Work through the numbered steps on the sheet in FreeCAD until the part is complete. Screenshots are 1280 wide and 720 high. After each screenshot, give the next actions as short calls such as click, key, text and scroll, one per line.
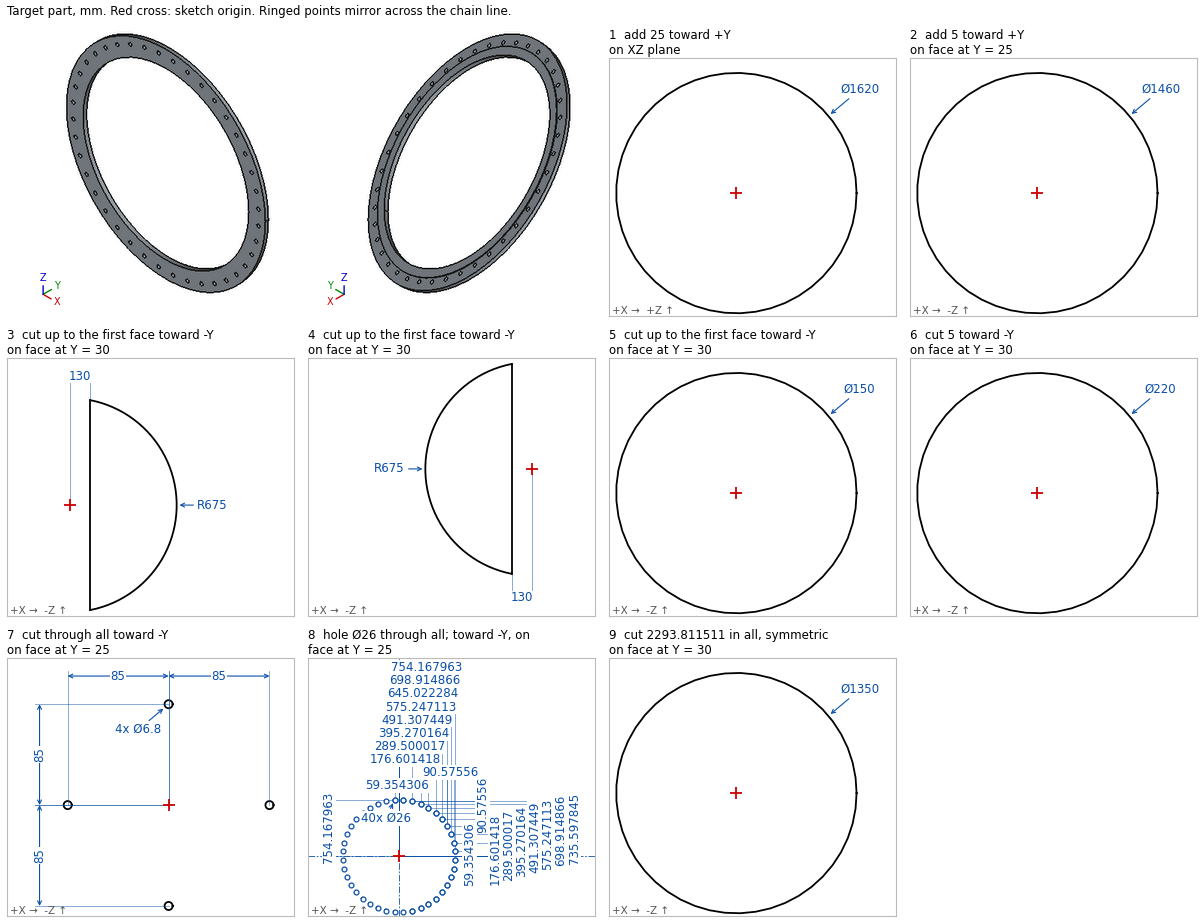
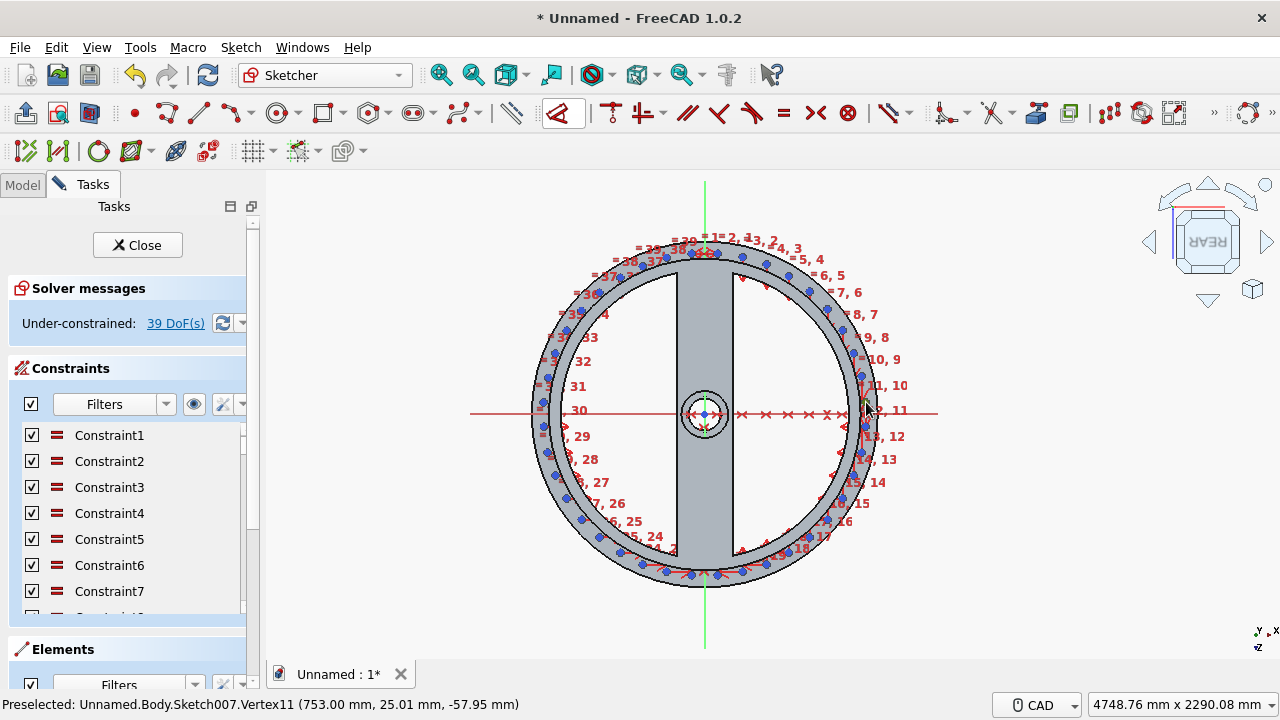
click(544, 402)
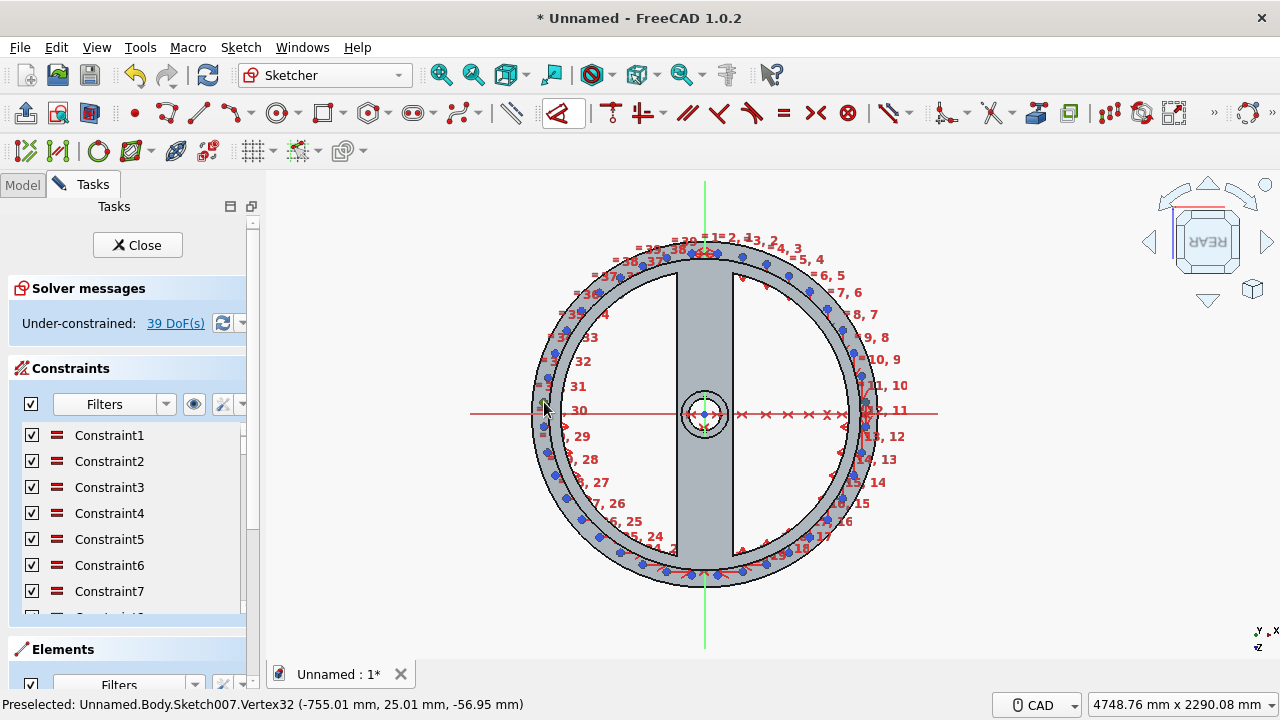
click(705, 507)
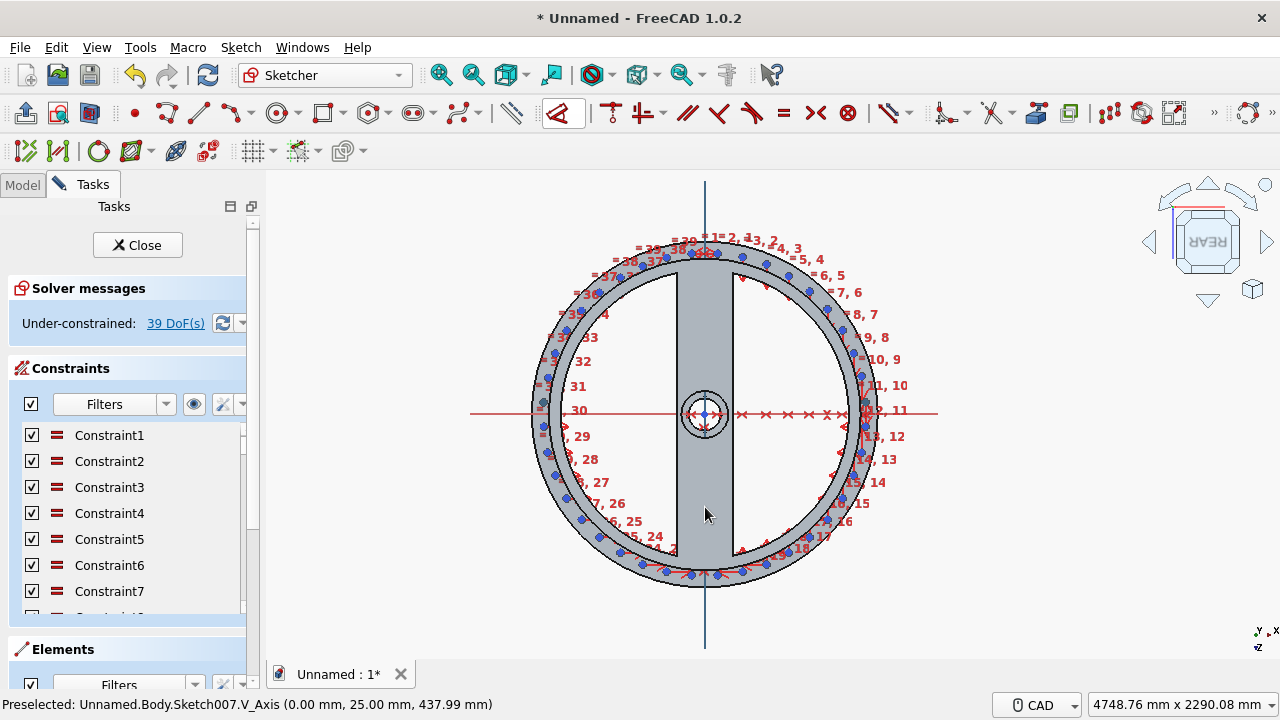
click(816, 114)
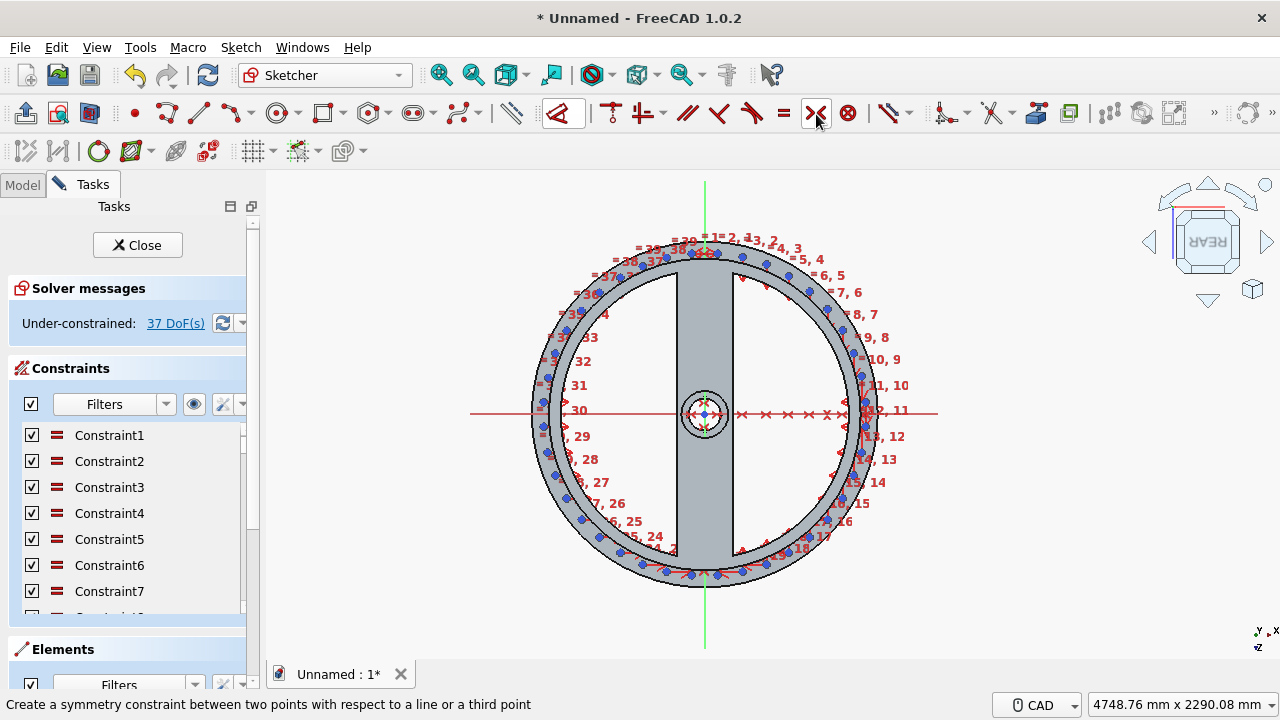
click(862, 376)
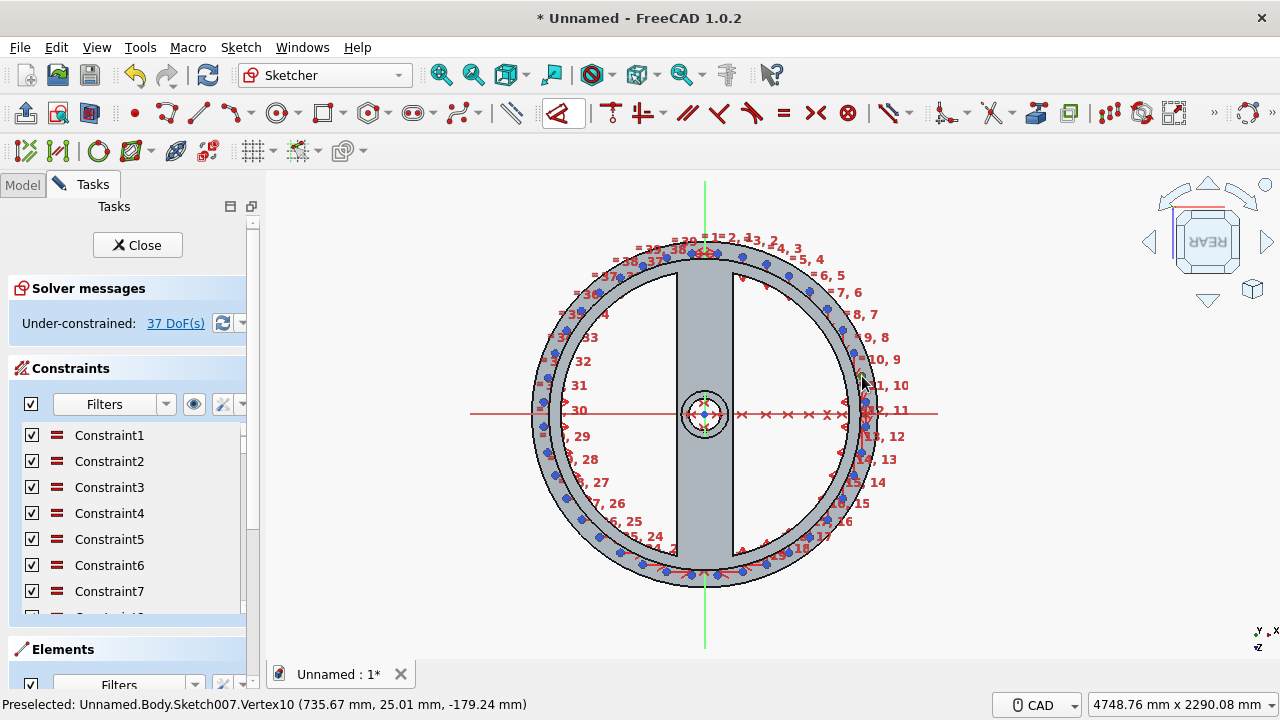
click(548, 378)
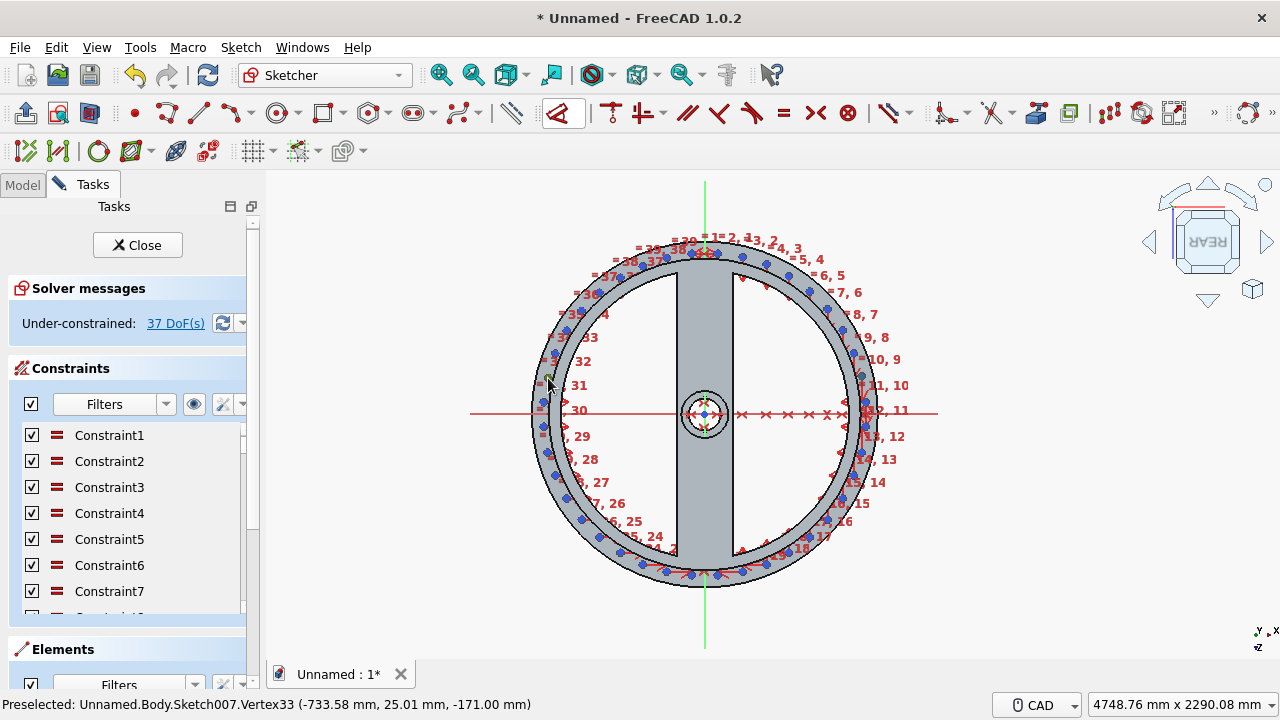
click(705, 507)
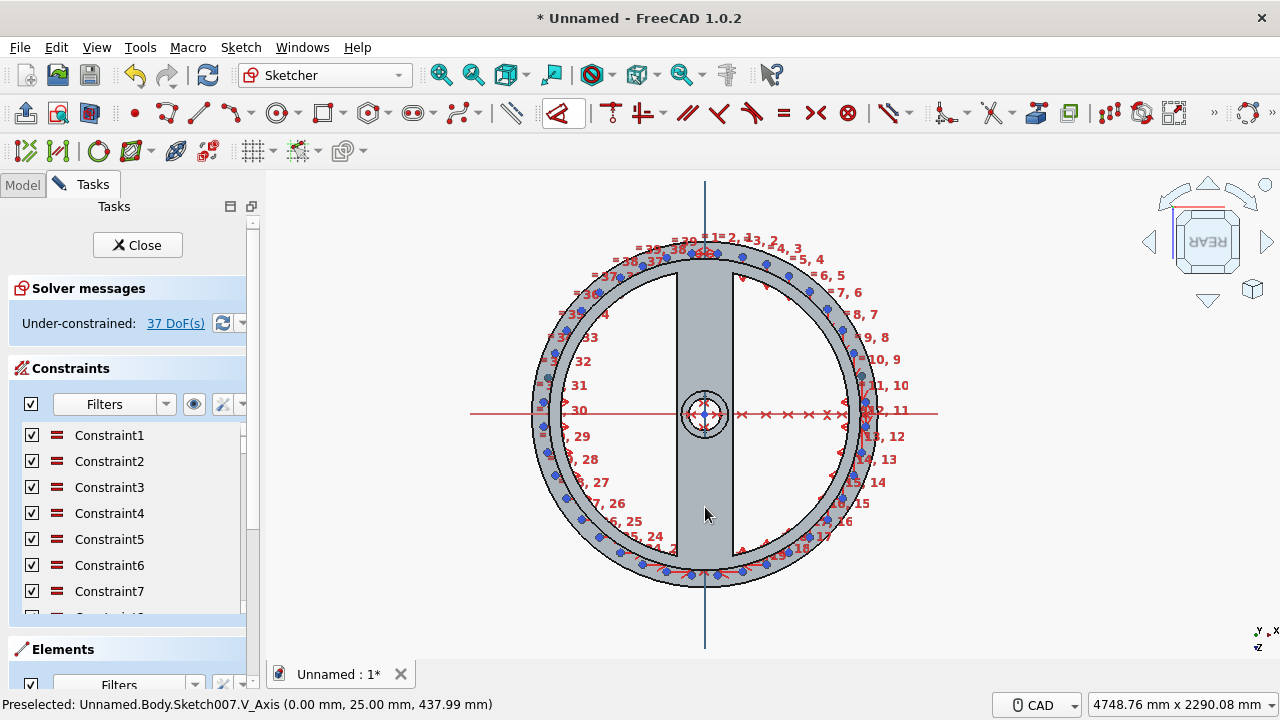
click(816, 114)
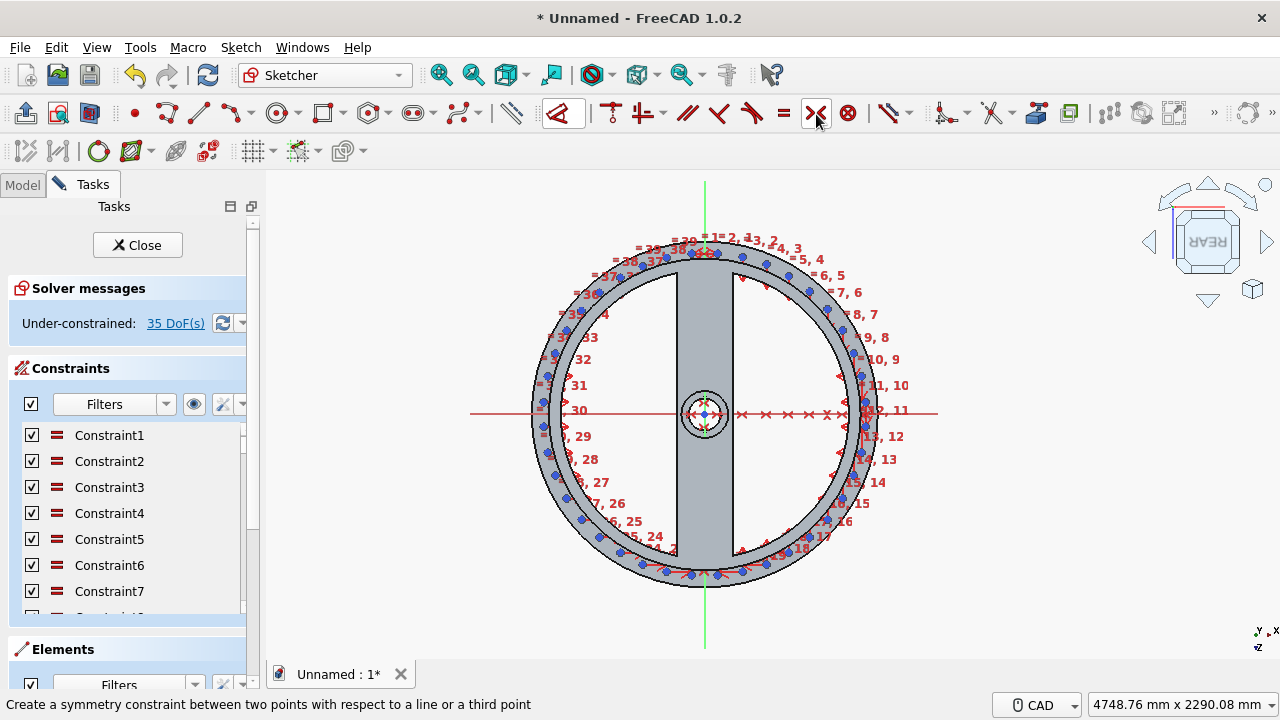
click(854, 353)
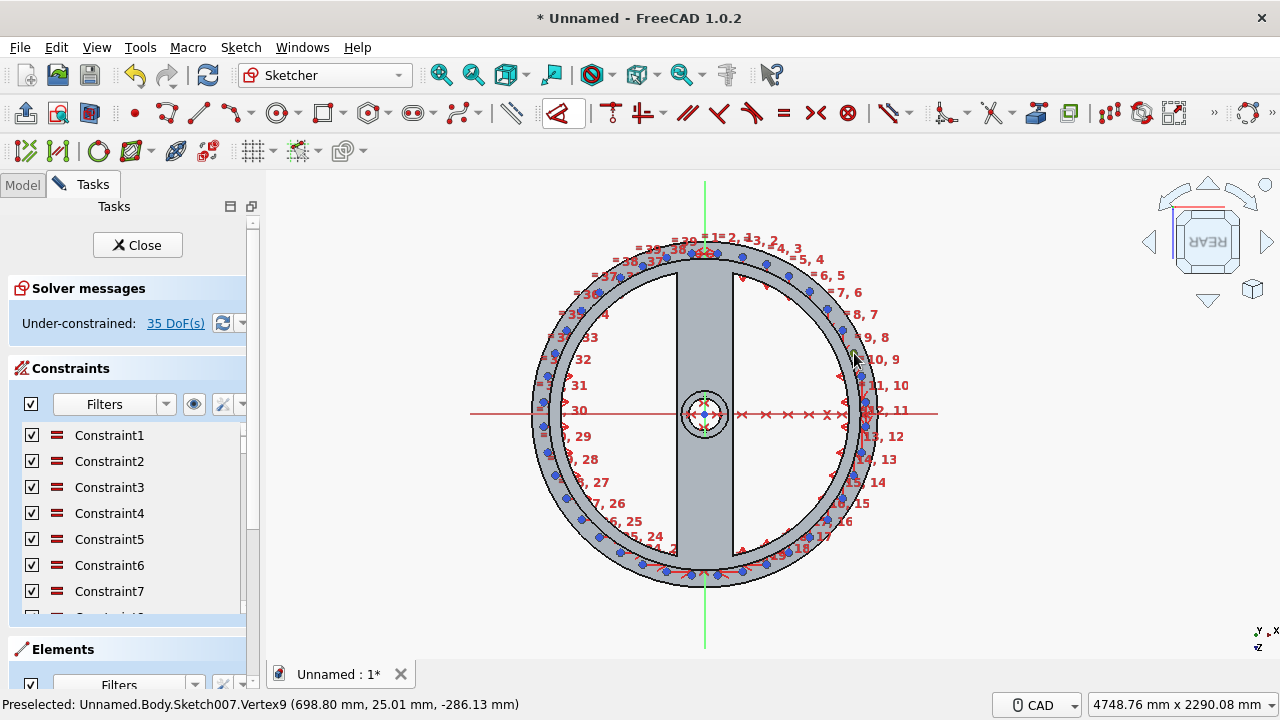
click(555, 354)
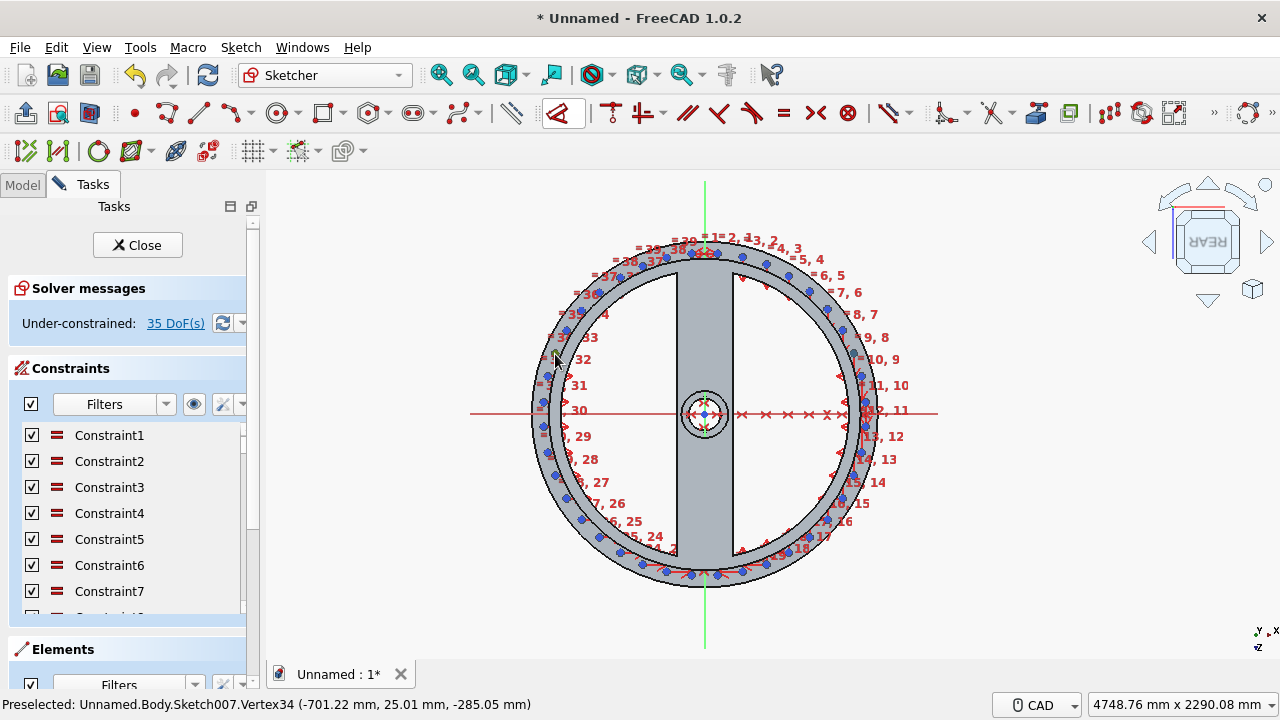
click(705, 507)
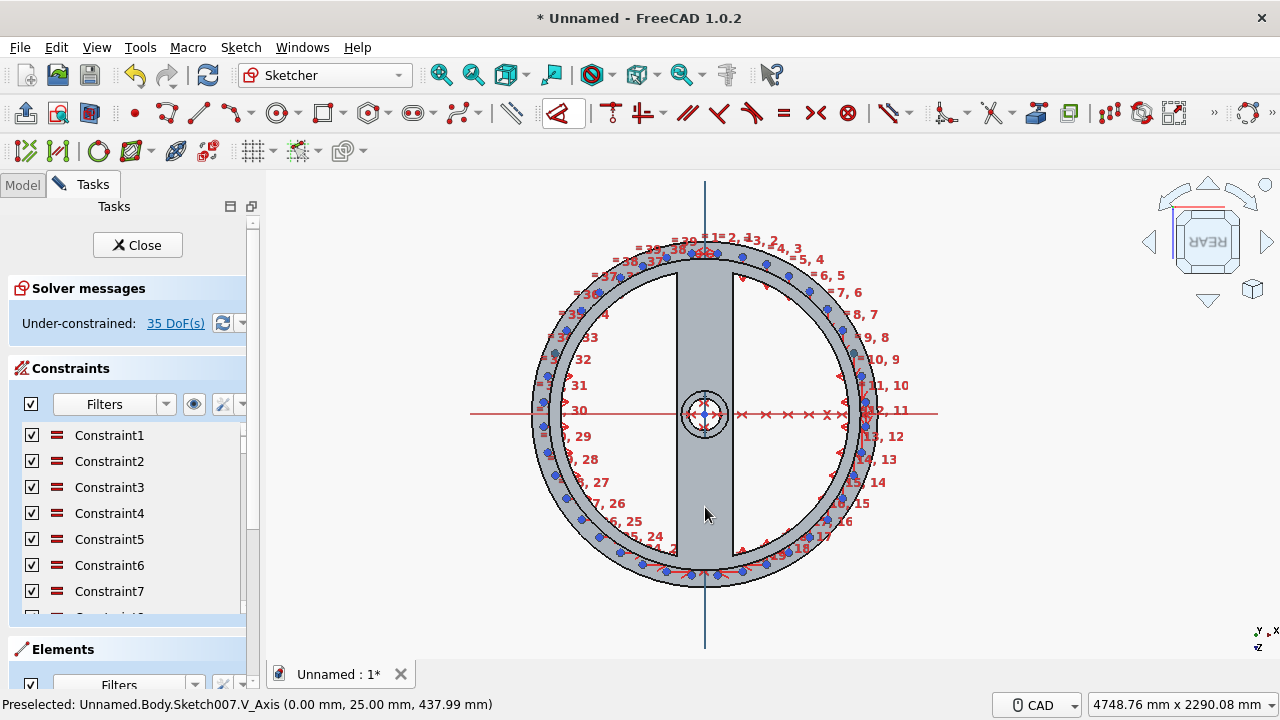
click(816, 114)